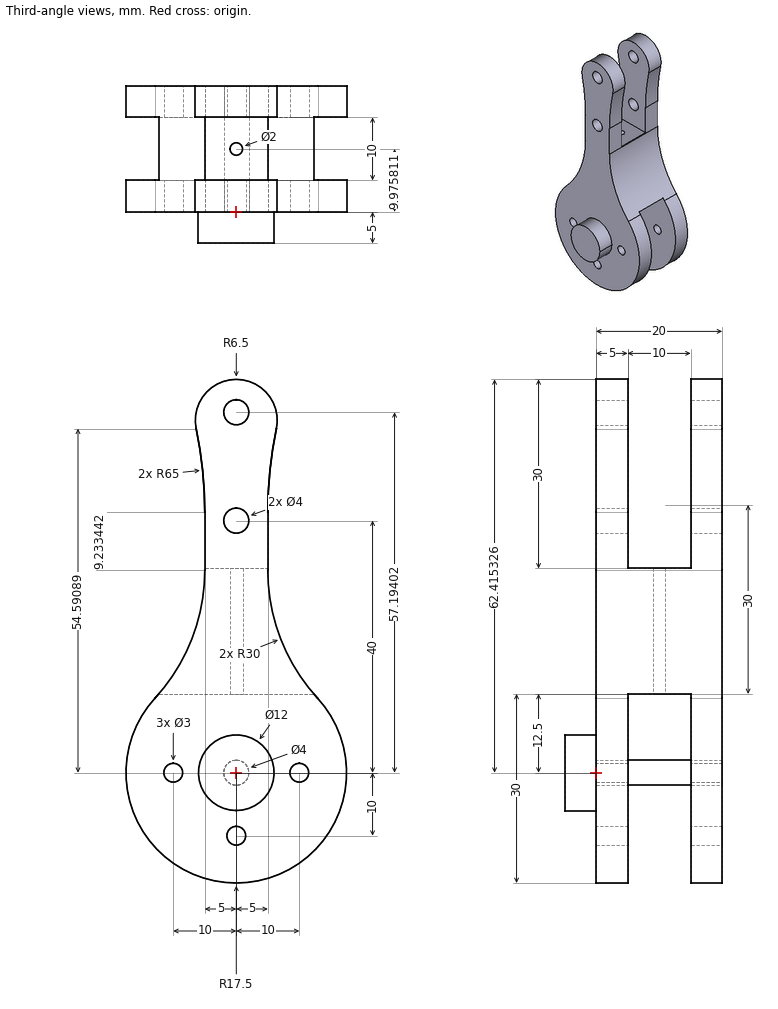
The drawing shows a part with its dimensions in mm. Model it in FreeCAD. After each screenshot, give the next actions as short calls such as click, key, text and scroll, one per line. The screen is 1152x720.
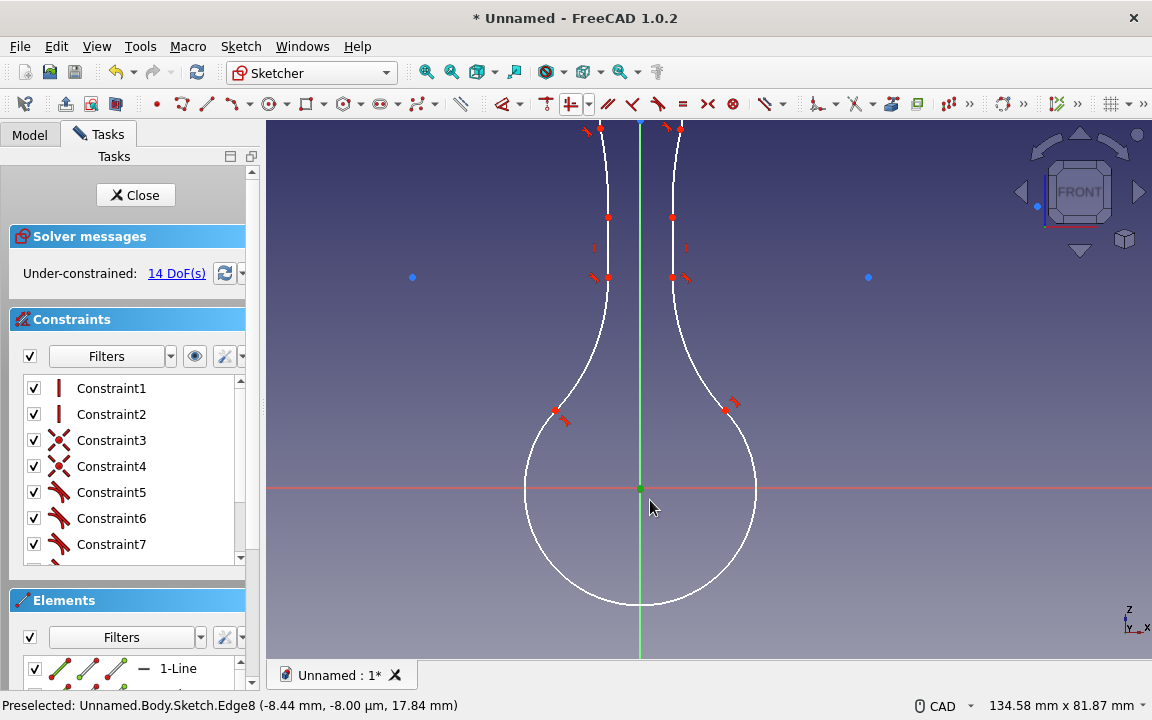
key(c)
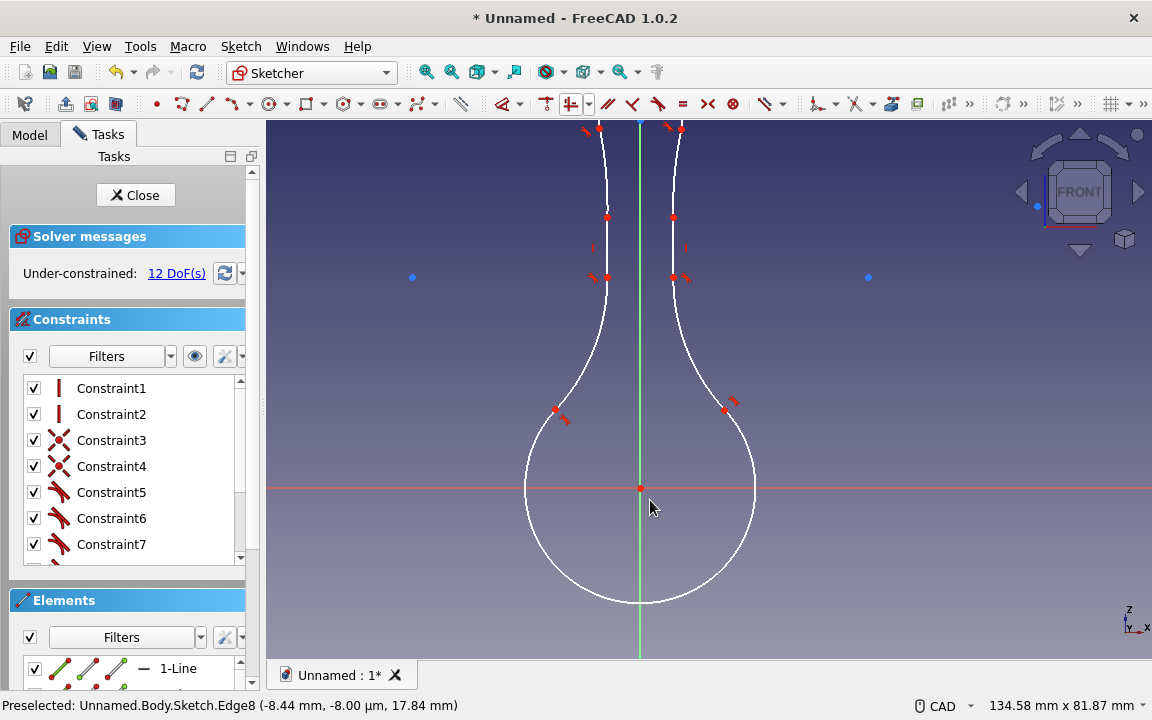
click(607, 191)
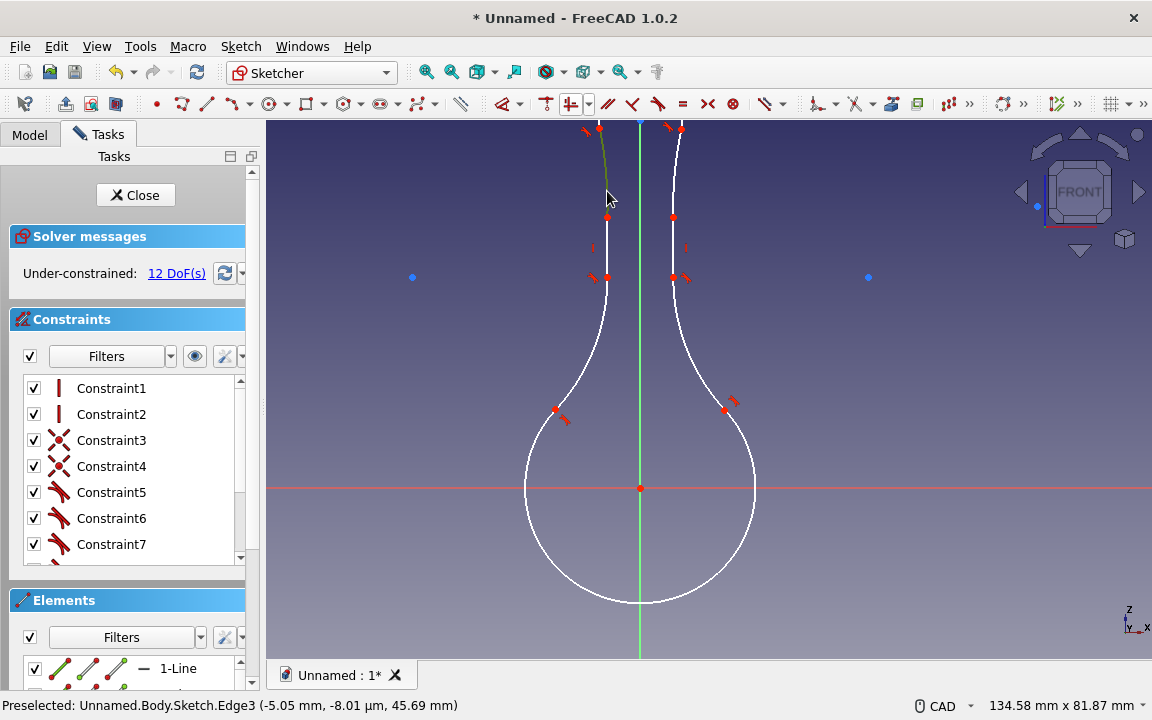
click(677, 156)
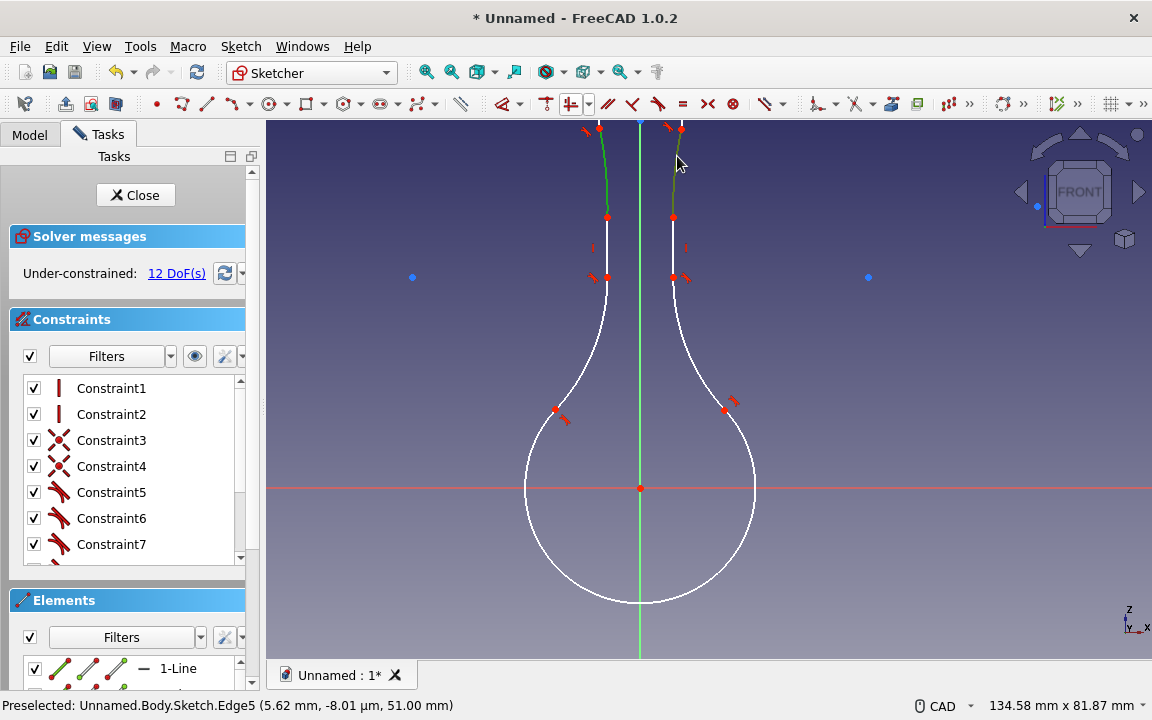
key(e)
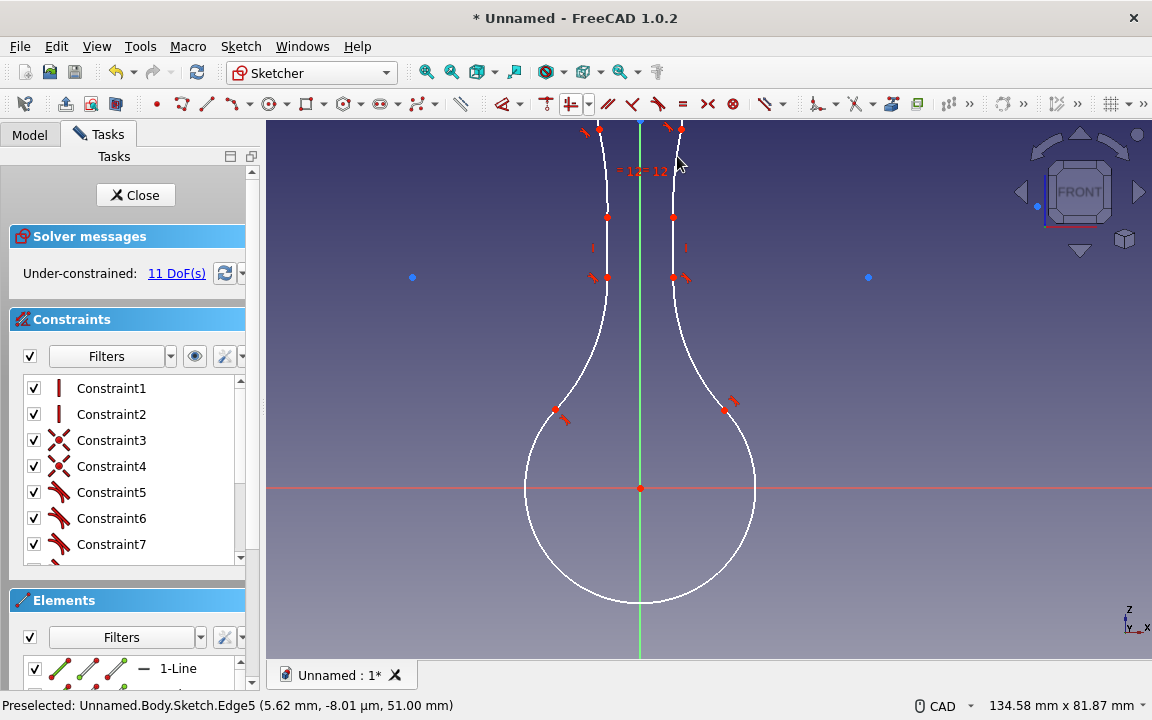
click(678, 321)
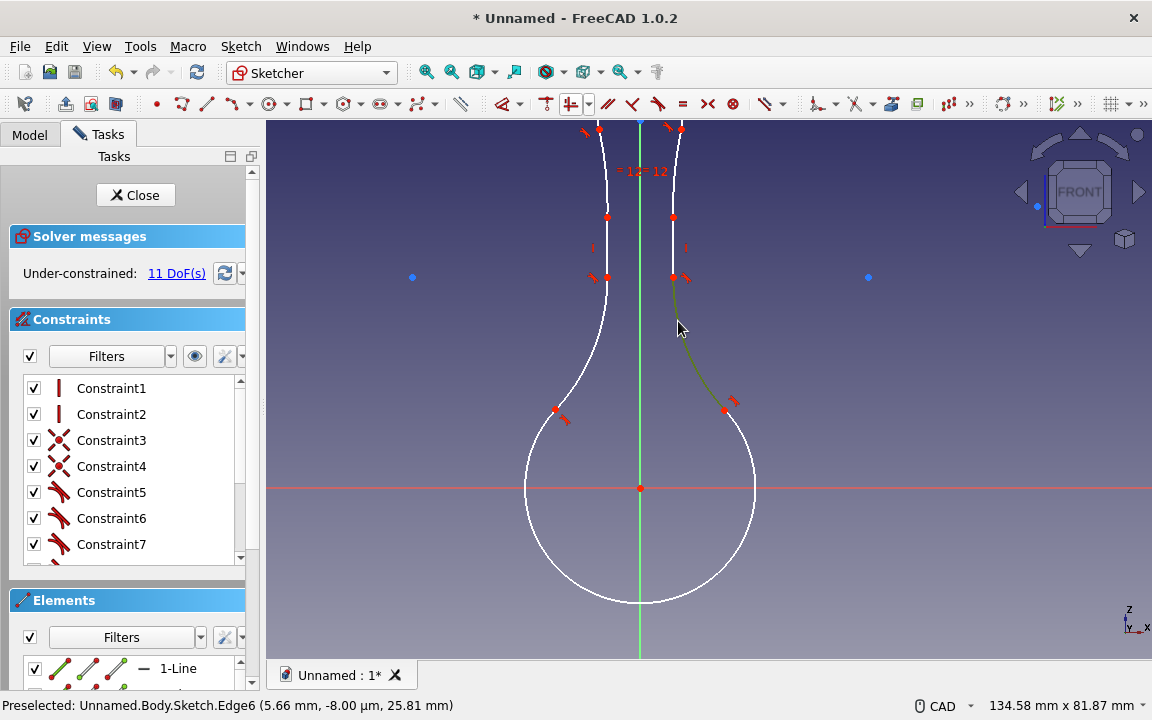
click(581, 375)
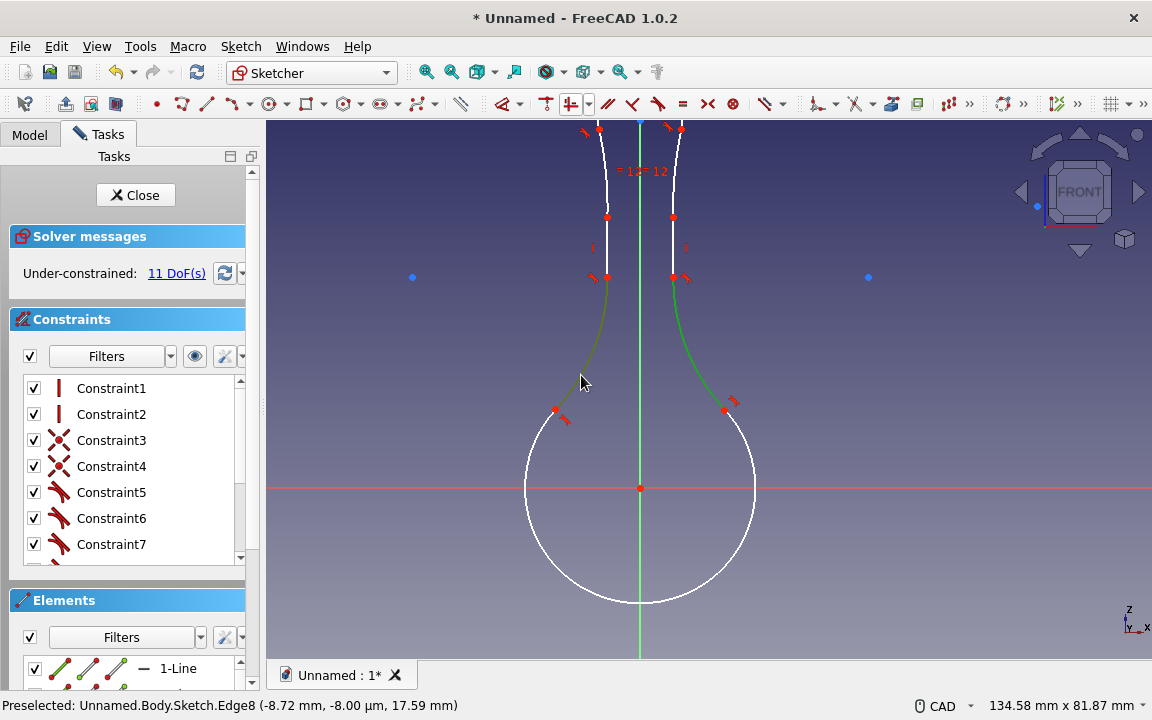
click(683, 104)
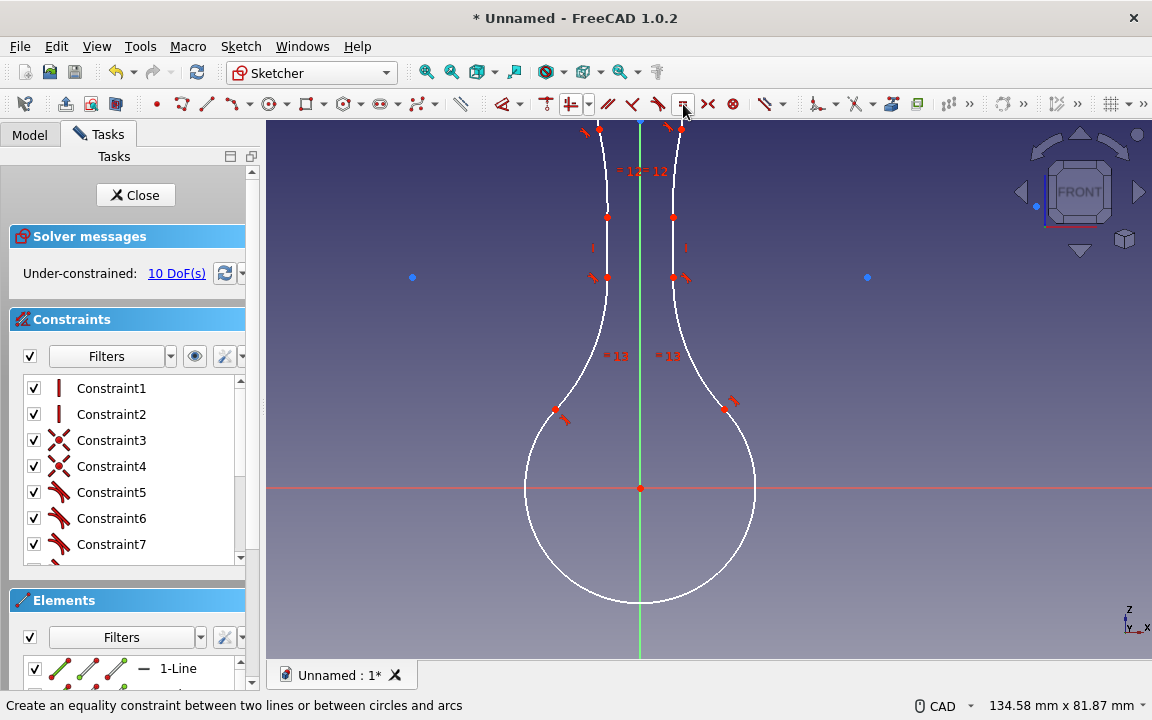
scroll(641, 490, down, 2)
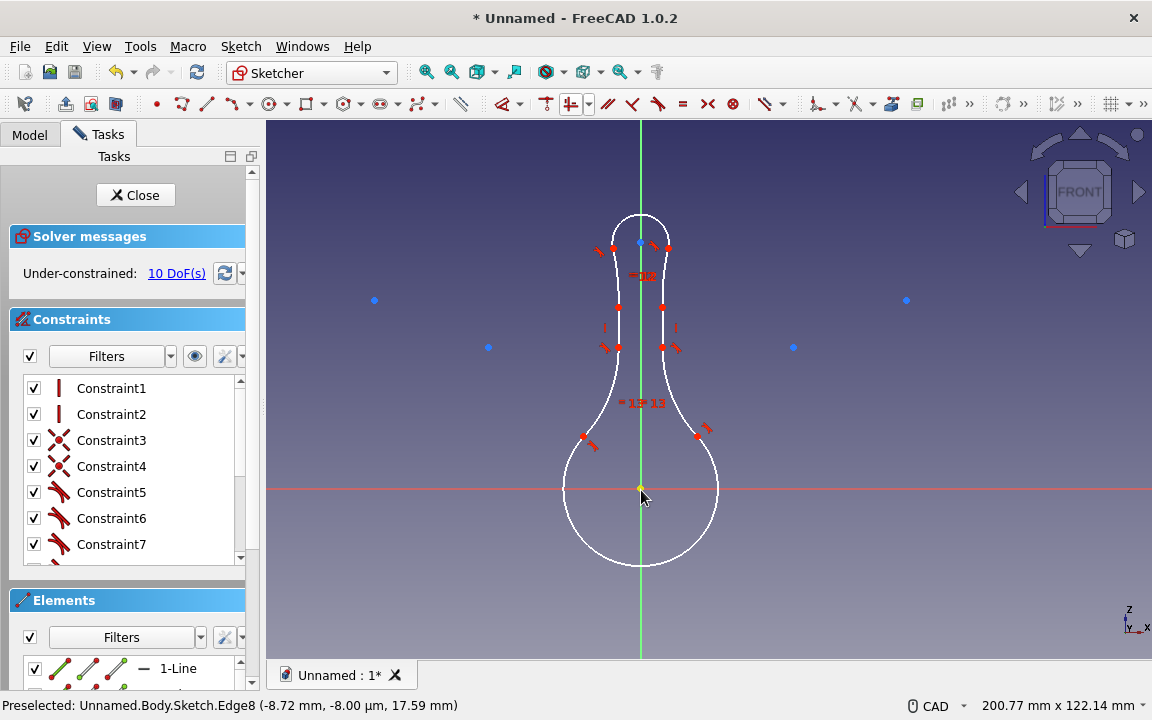
click(641, 243)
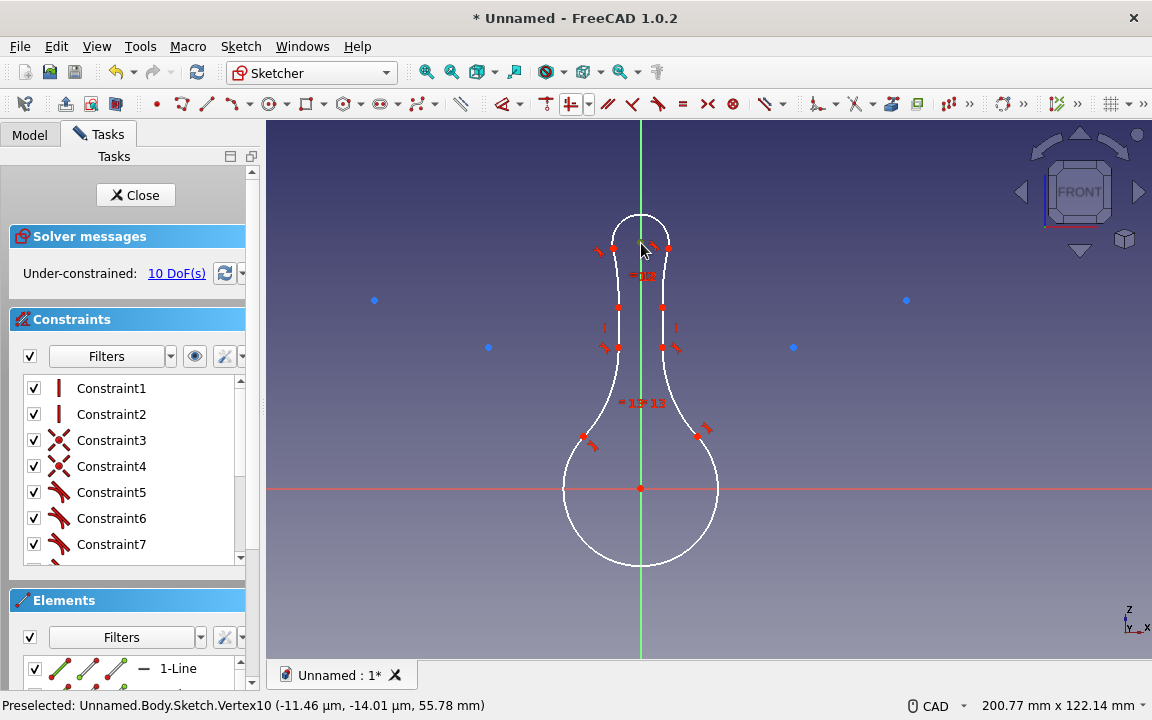
click(641, 596)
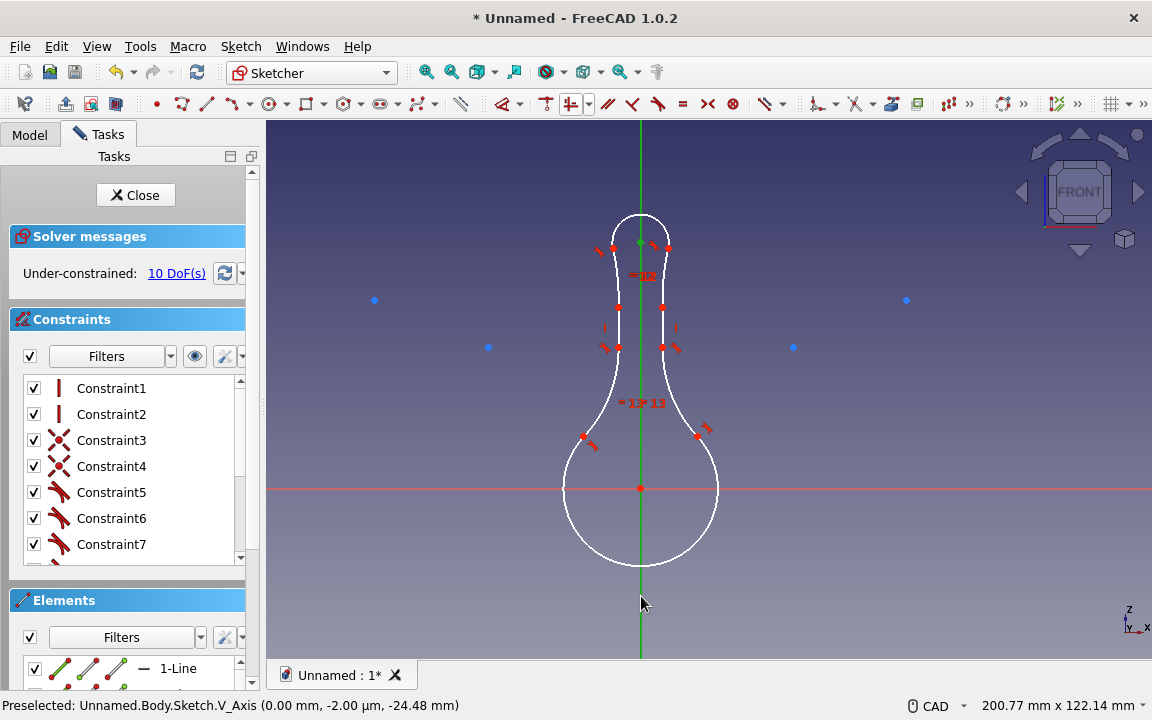
click(546, 104)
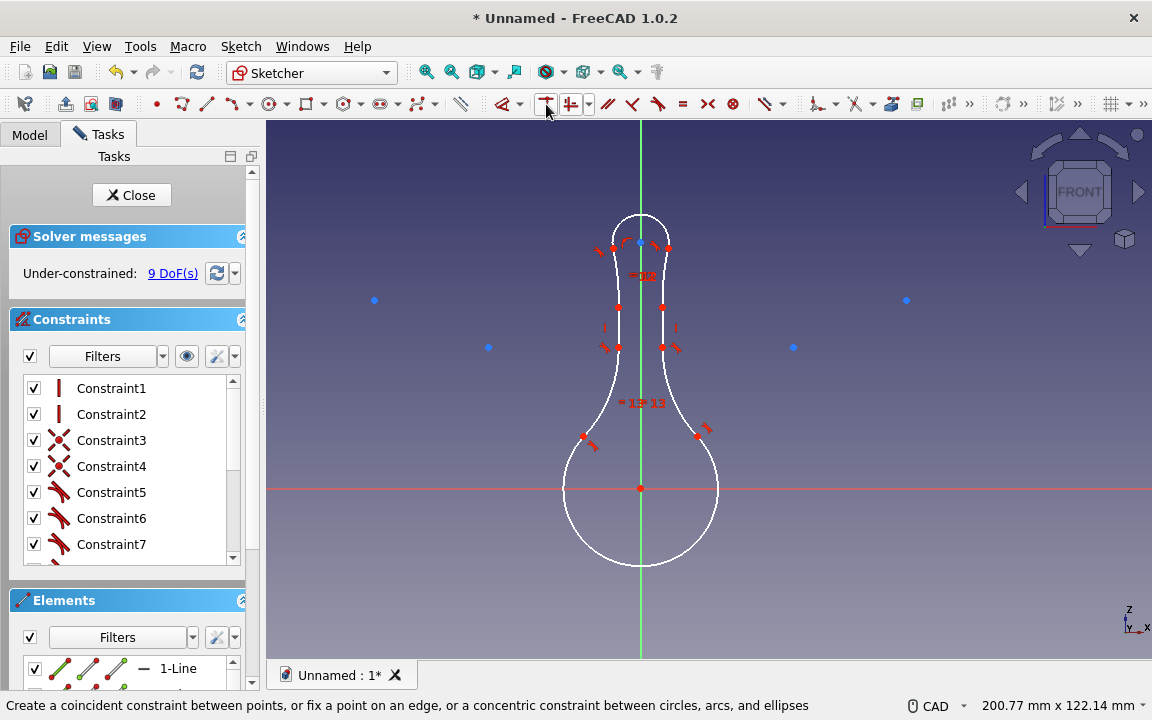
click(619, 290)